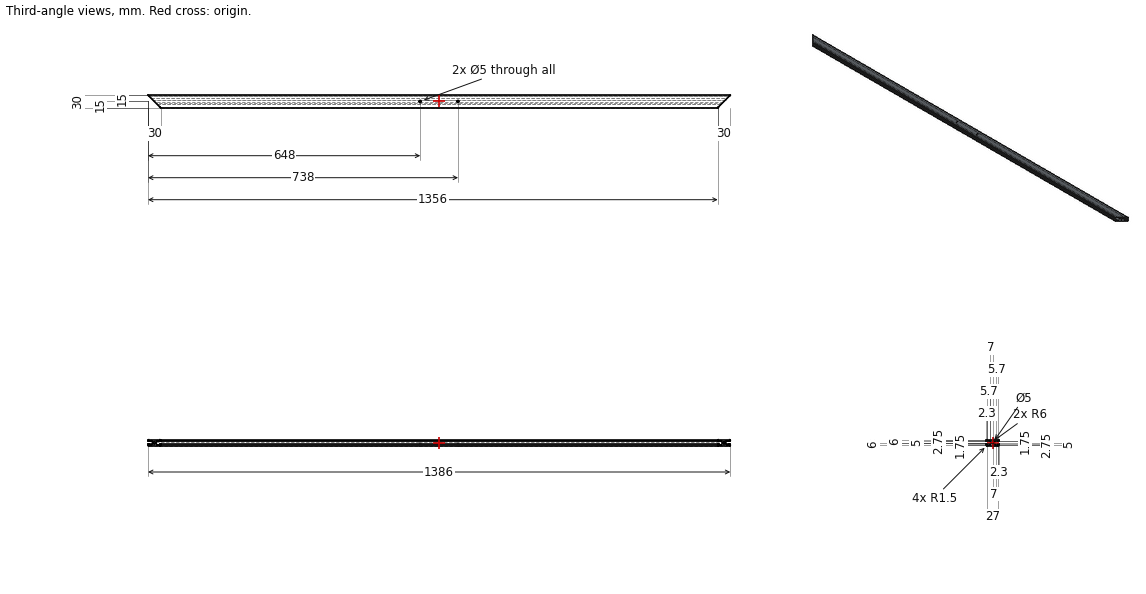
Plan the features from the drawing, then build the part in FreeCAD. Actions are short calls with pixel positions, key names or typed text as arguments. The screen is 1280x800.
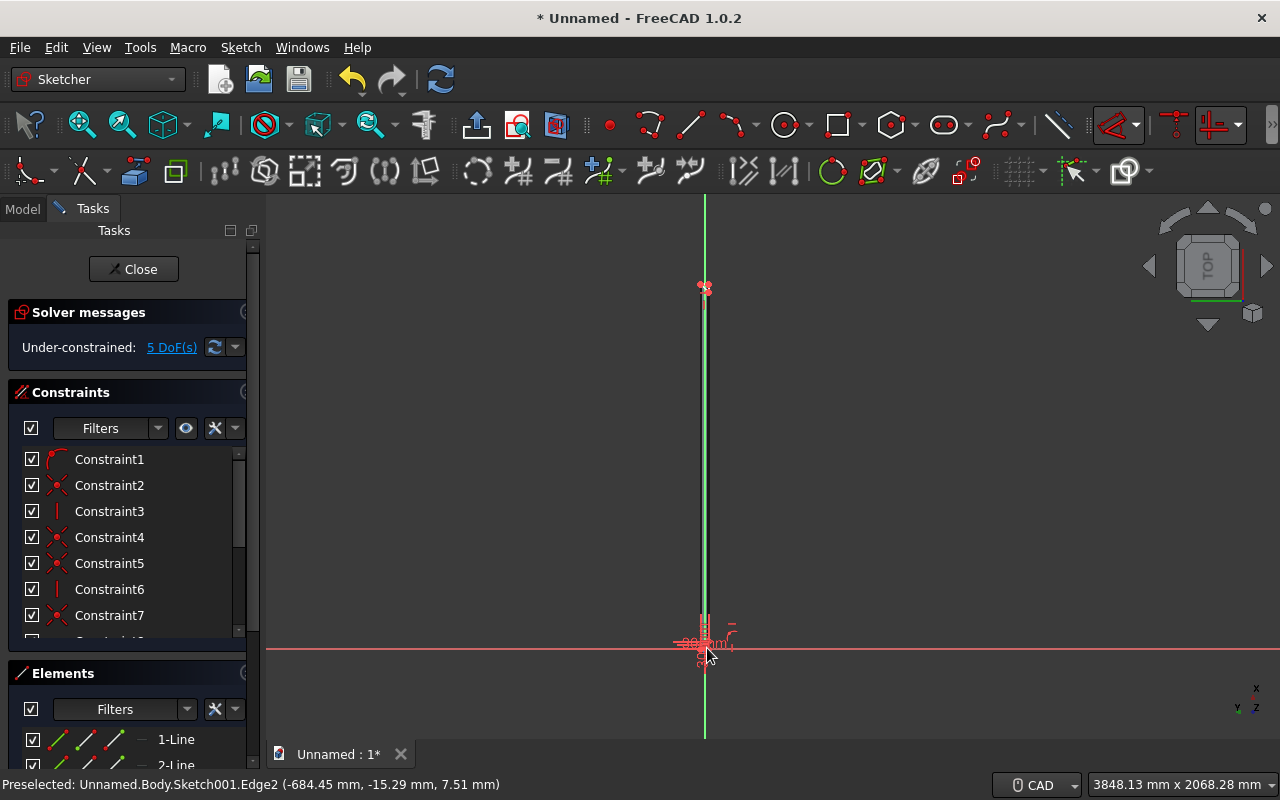
scroll(709, 290, up, 11)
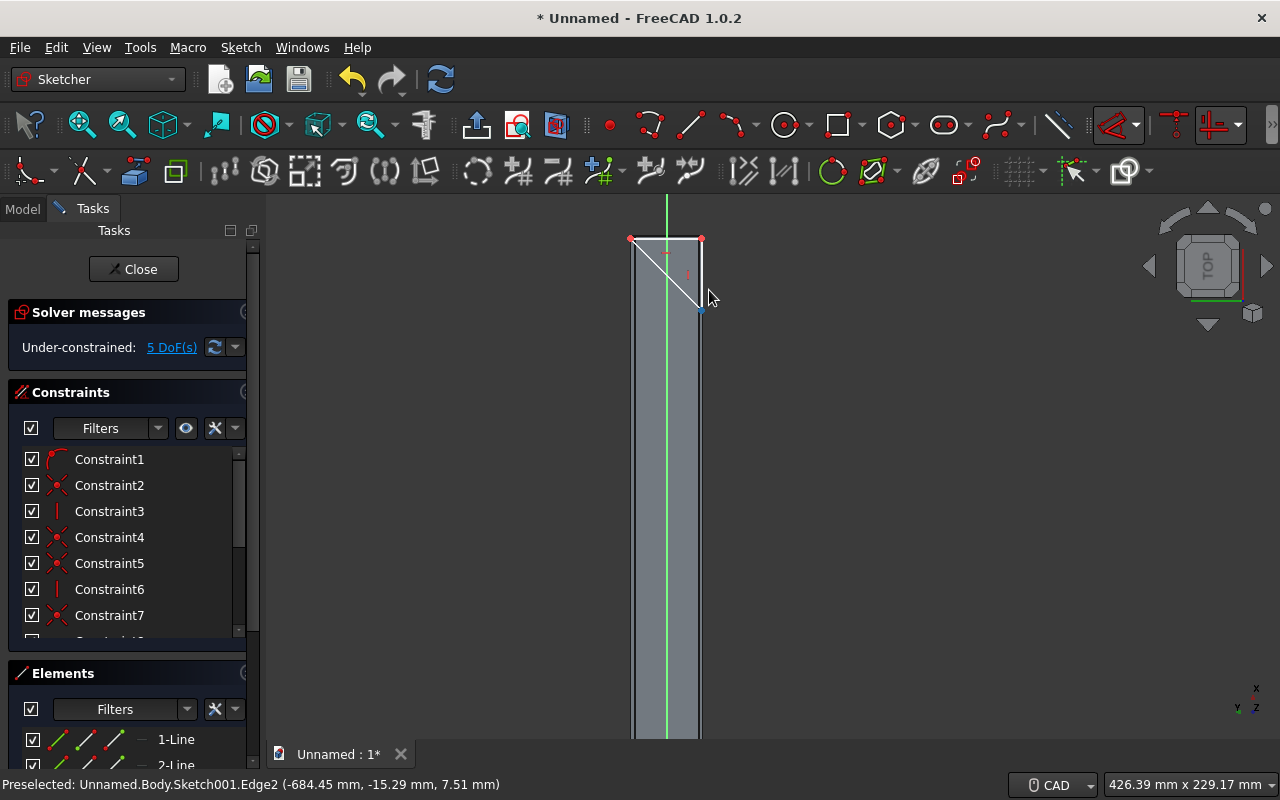
click(702, 289)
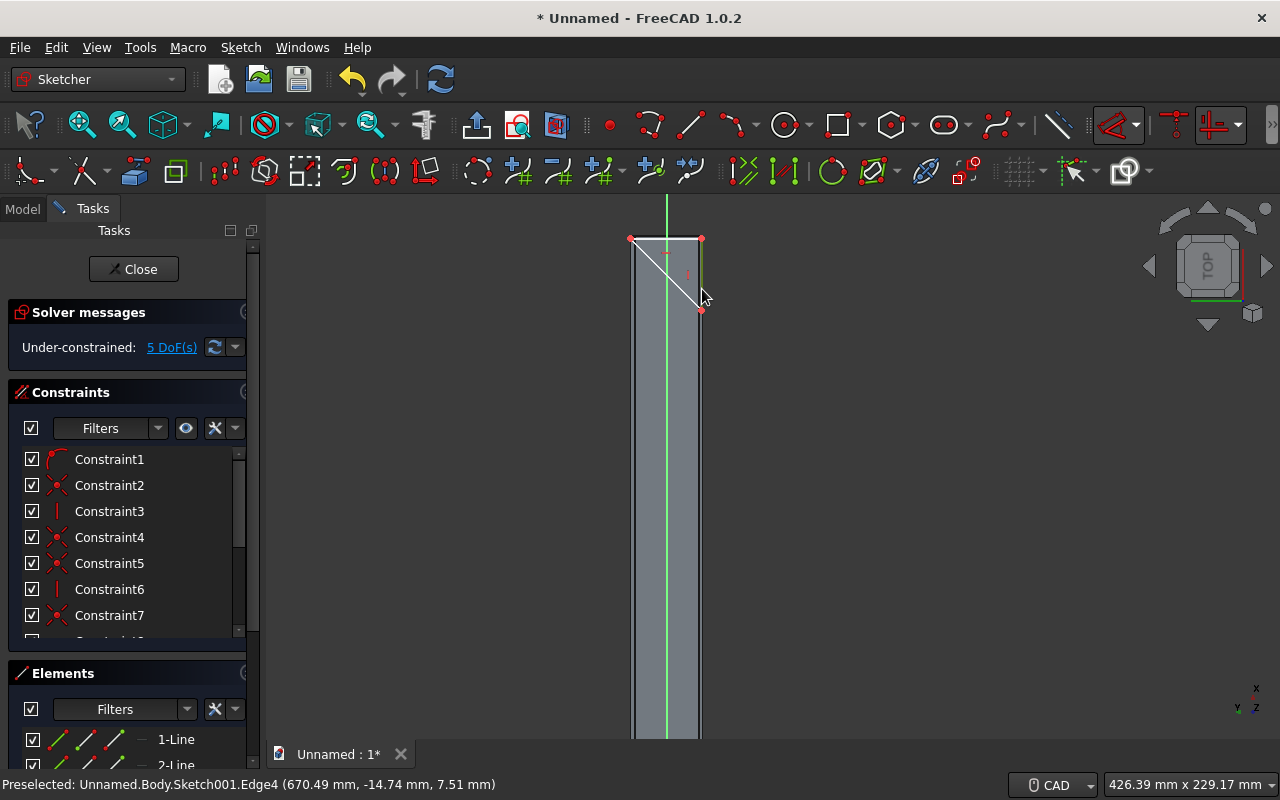
key(i)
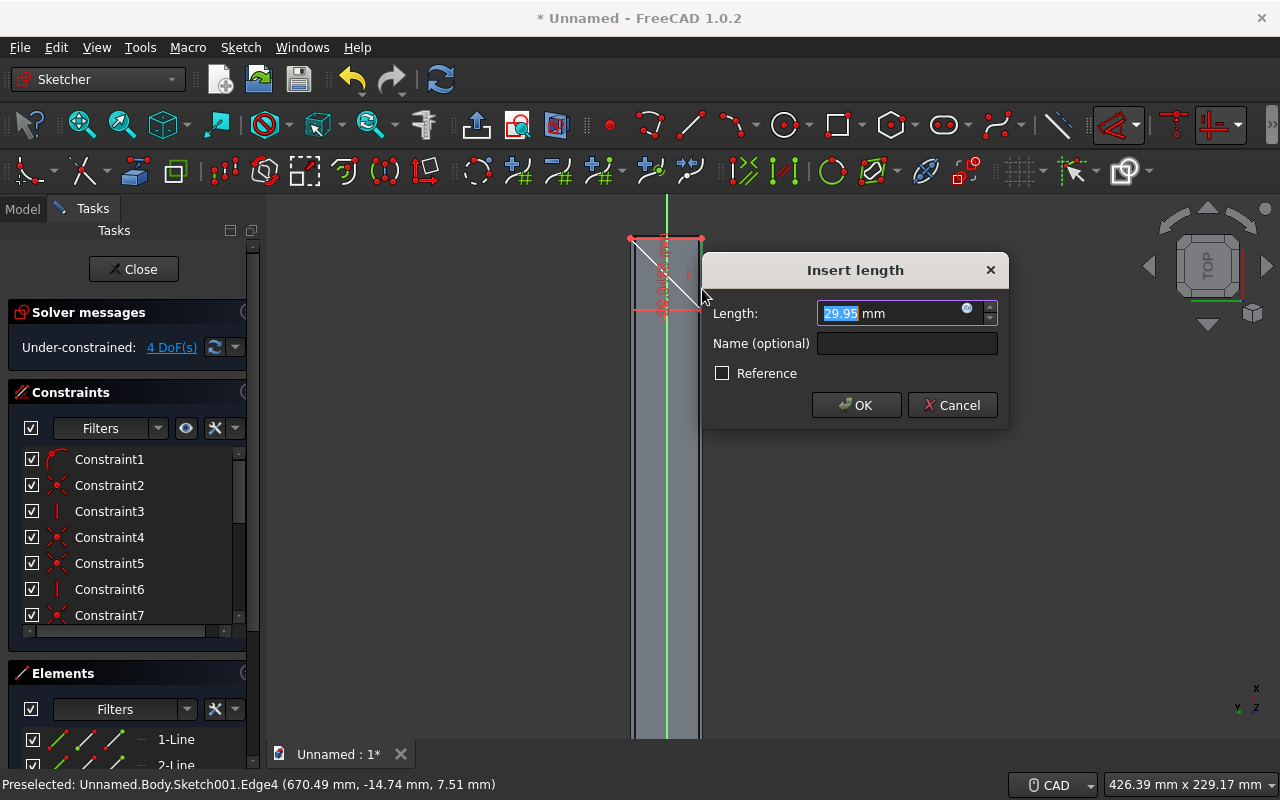
text(30)
key(Return)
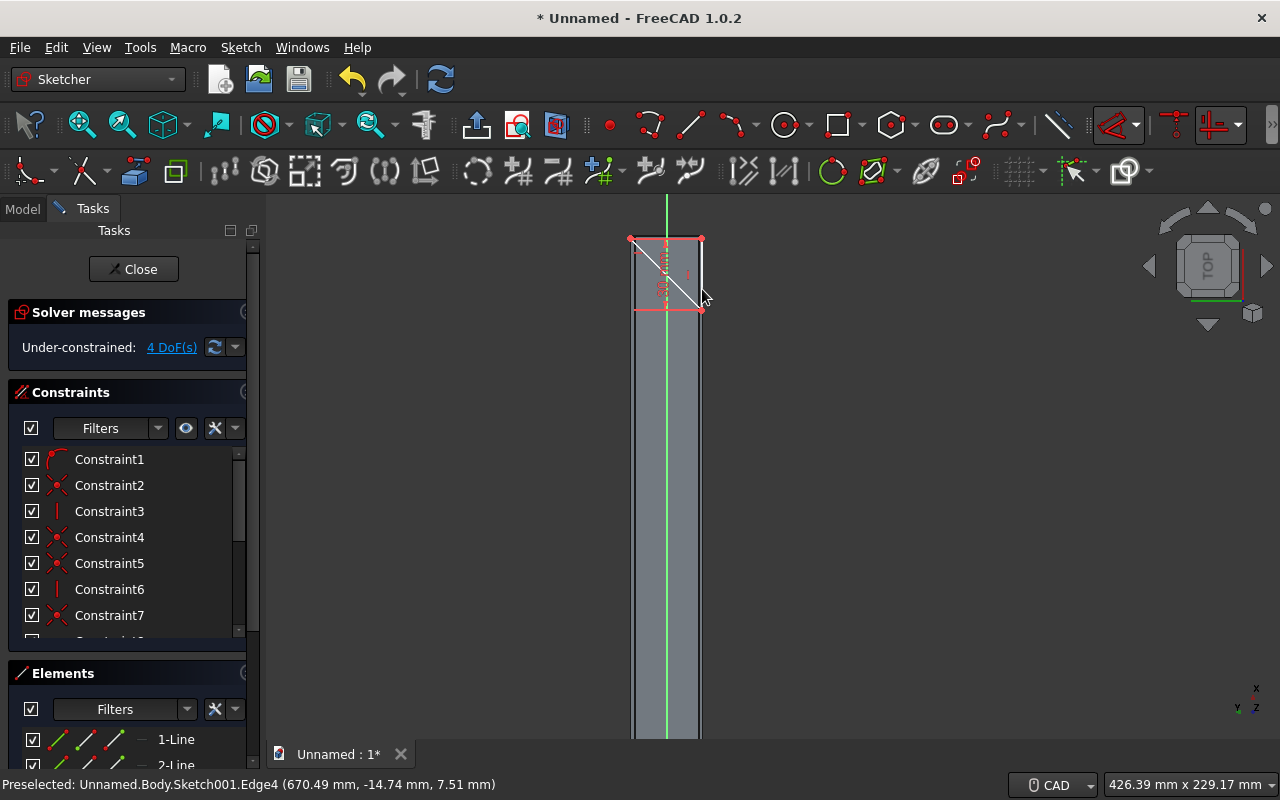
click(680, 239)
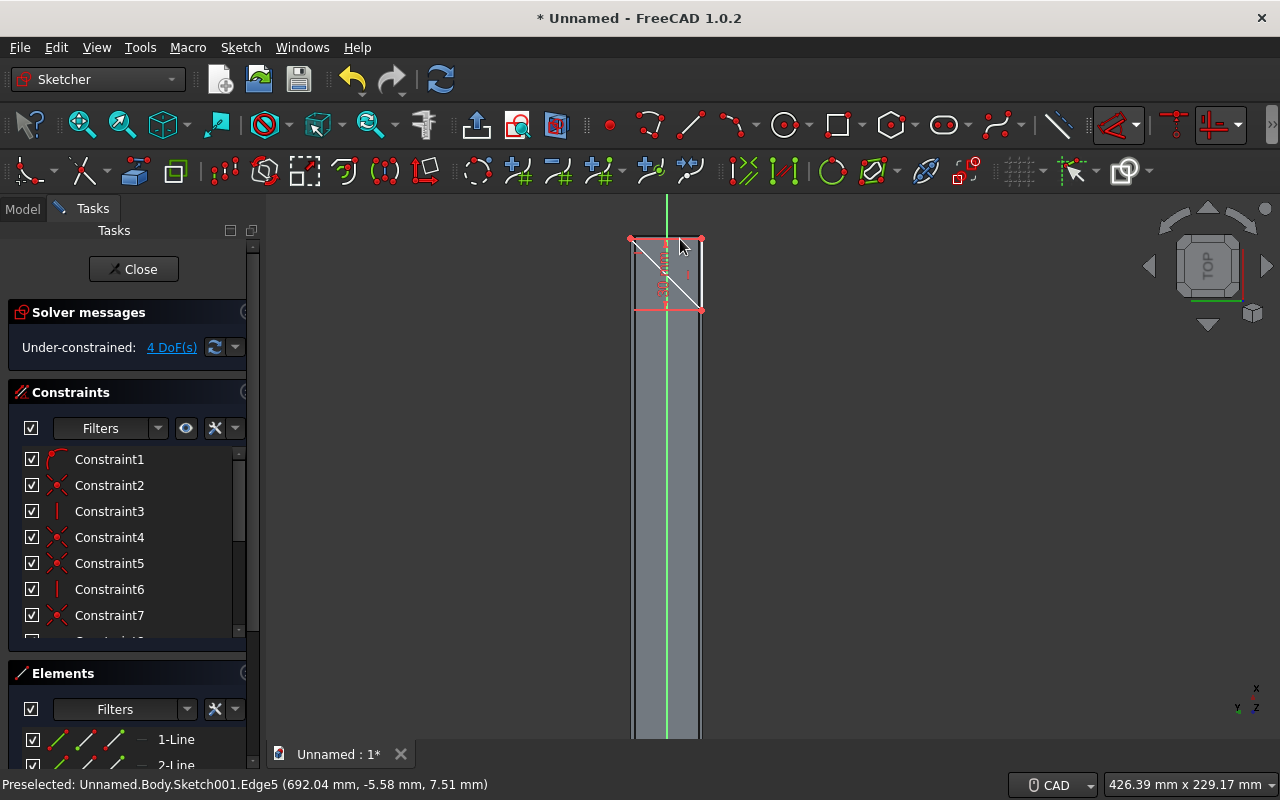
key(l)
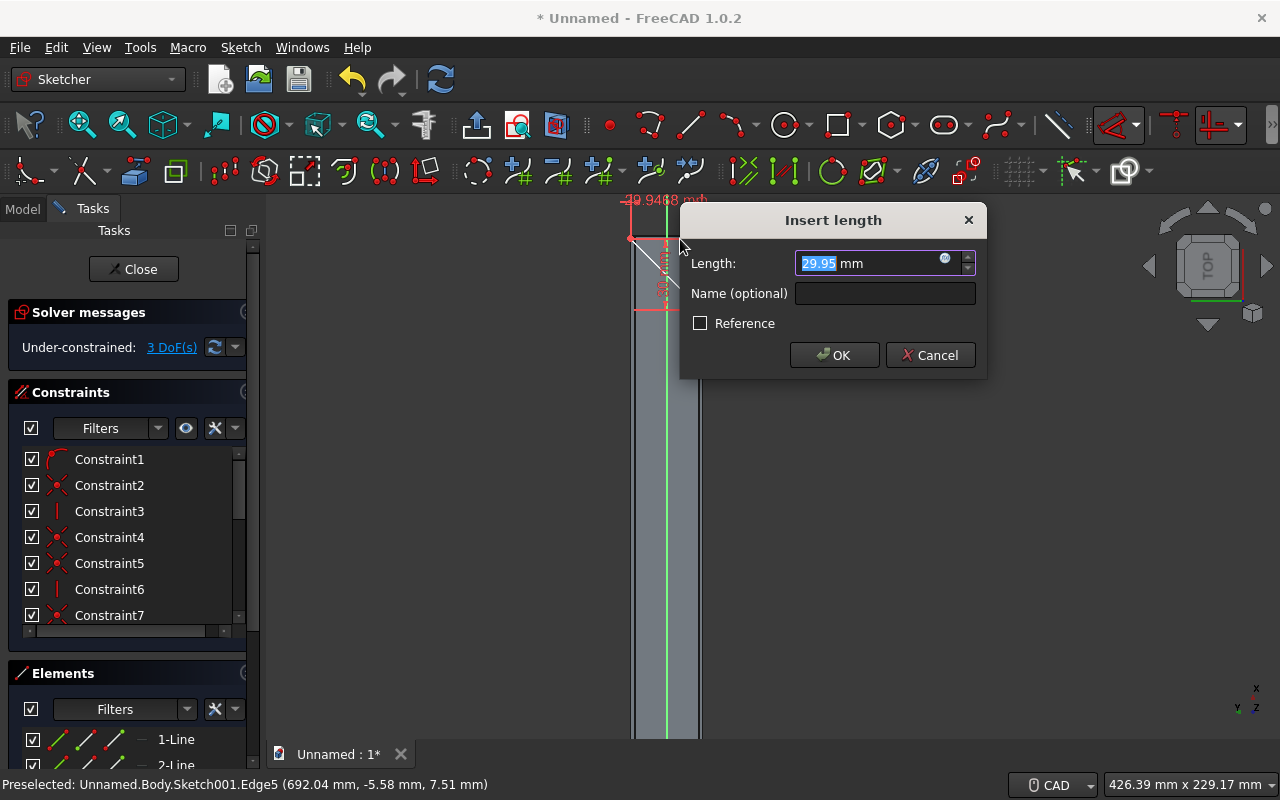
text(30)
key(Return)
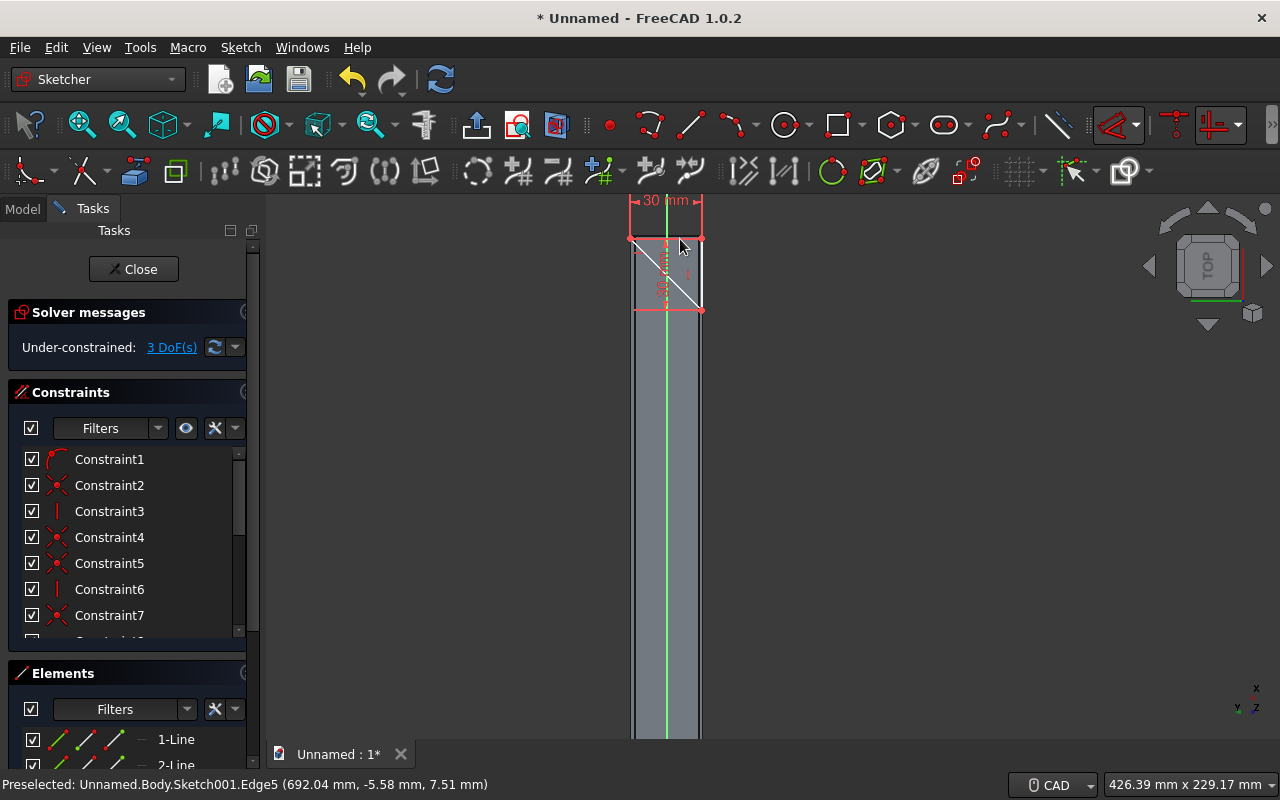
scroll(709, 290, down, 11)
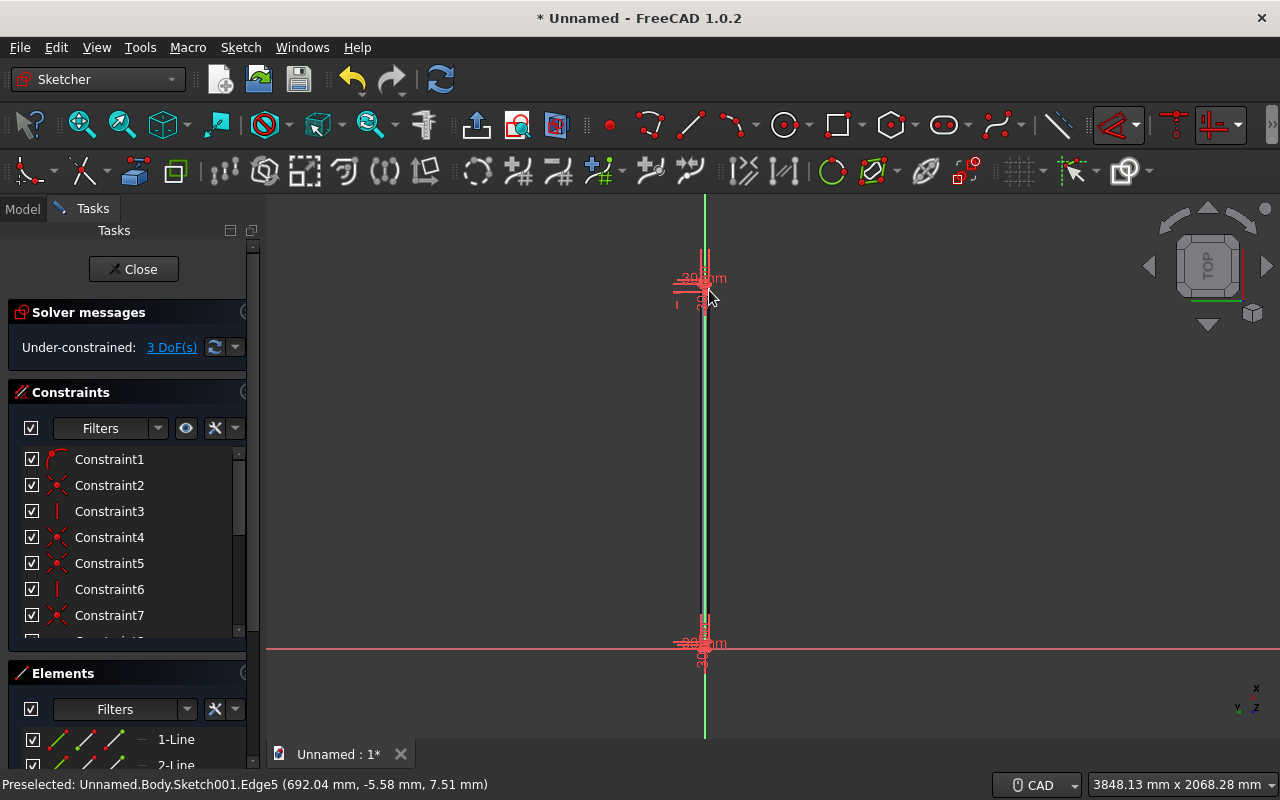
scroll(701, 649, up, 12)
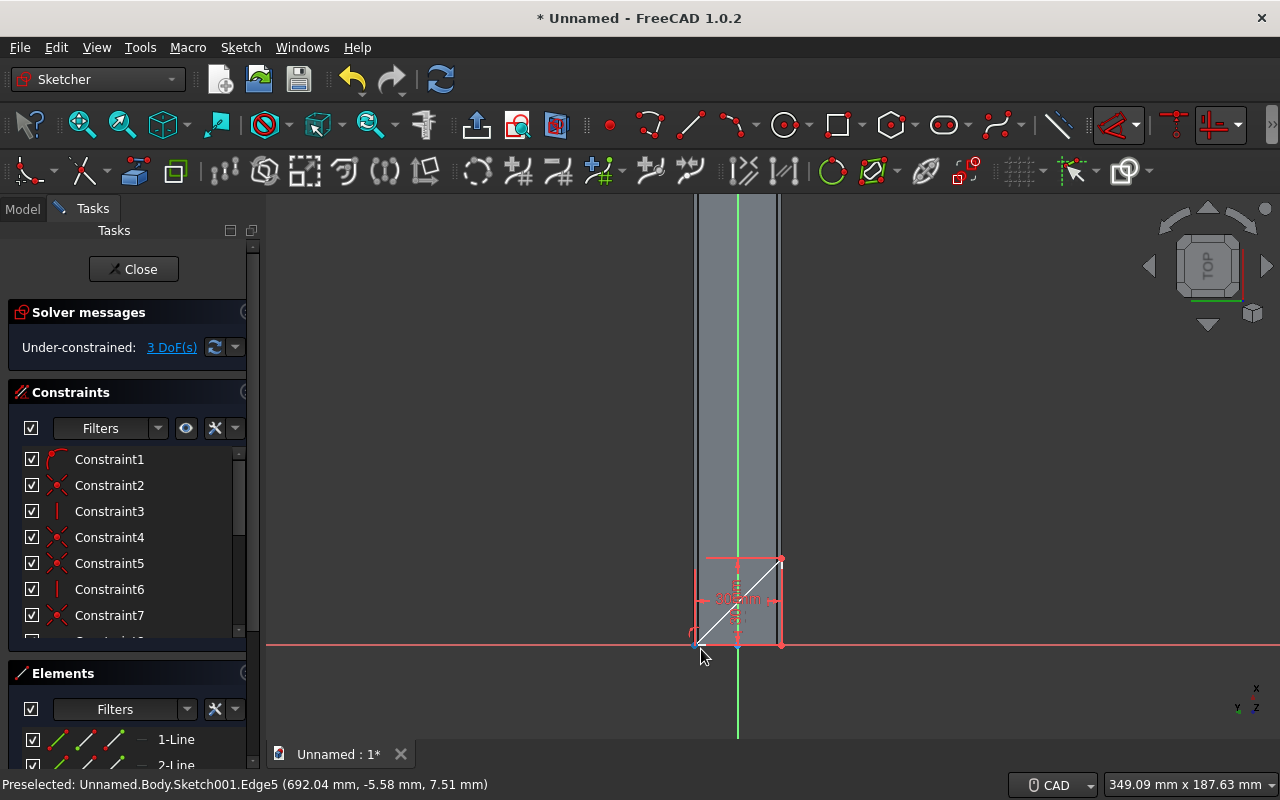
click(695, 645)